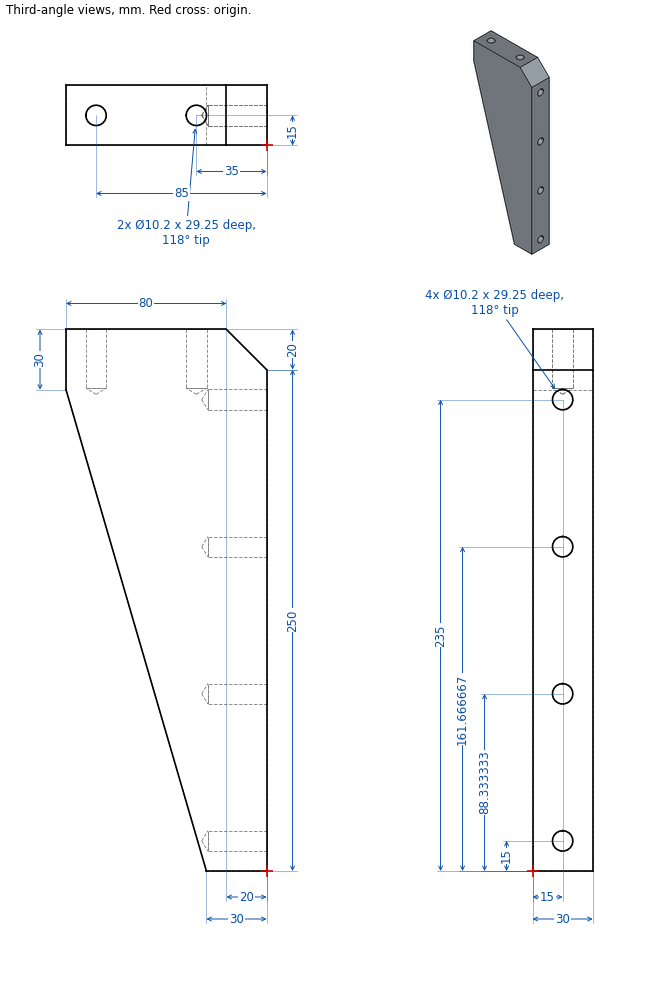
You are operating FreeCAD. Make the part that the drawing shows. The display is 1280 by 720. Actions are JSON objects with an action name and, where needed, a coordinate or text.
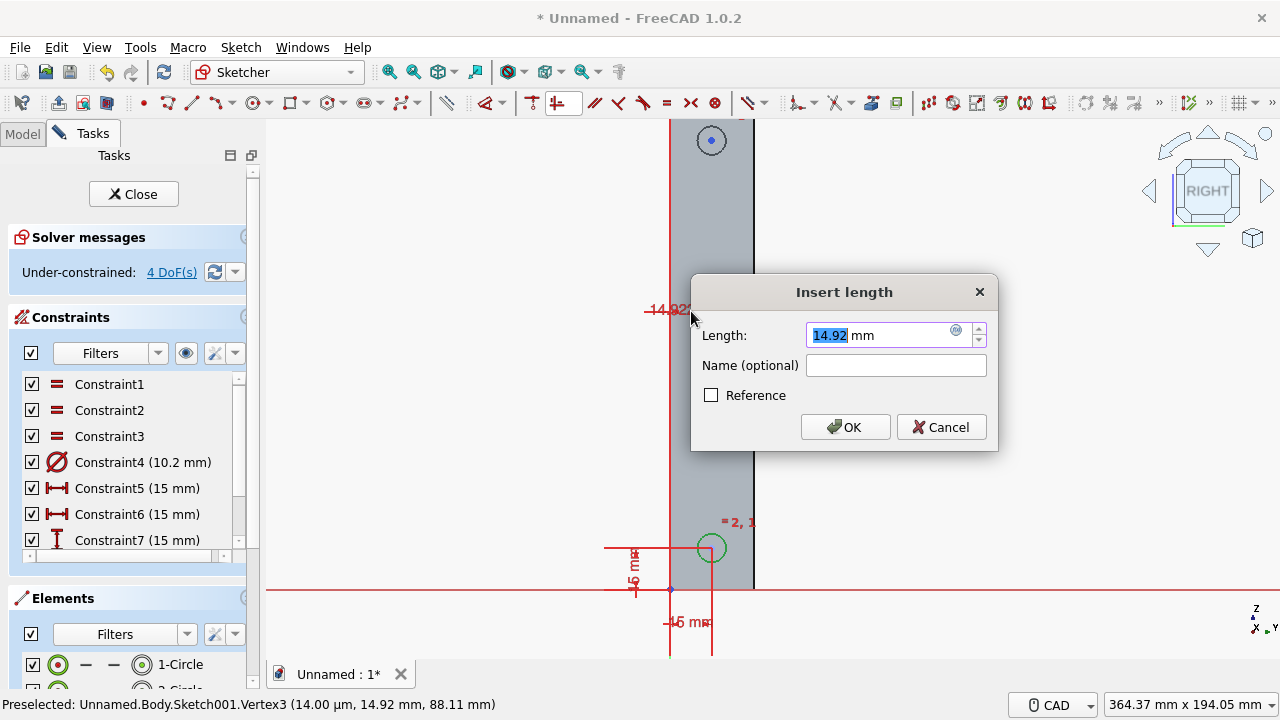
{"action": "type", "text": "15"}
{"action": "key", "text": "Return"}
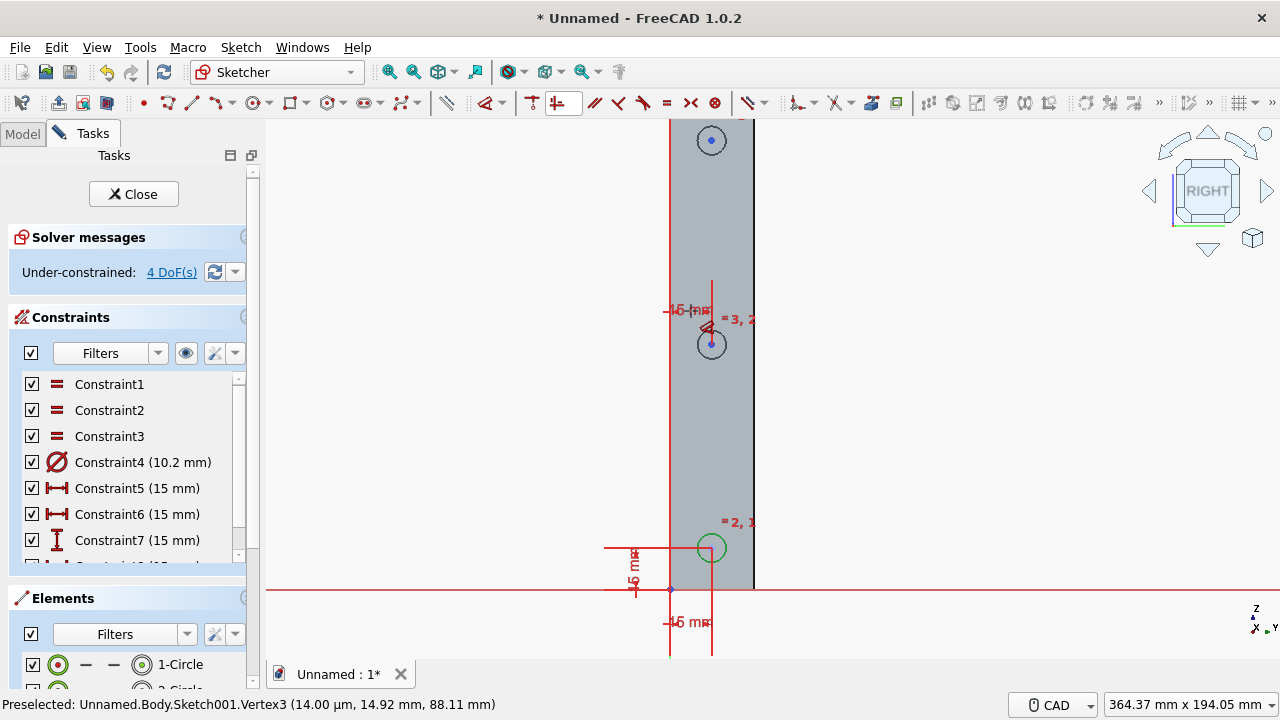
{"action": "scroll", "coordinate": [712, 551], "scroll_direction": "down", "scroll_amount": 3}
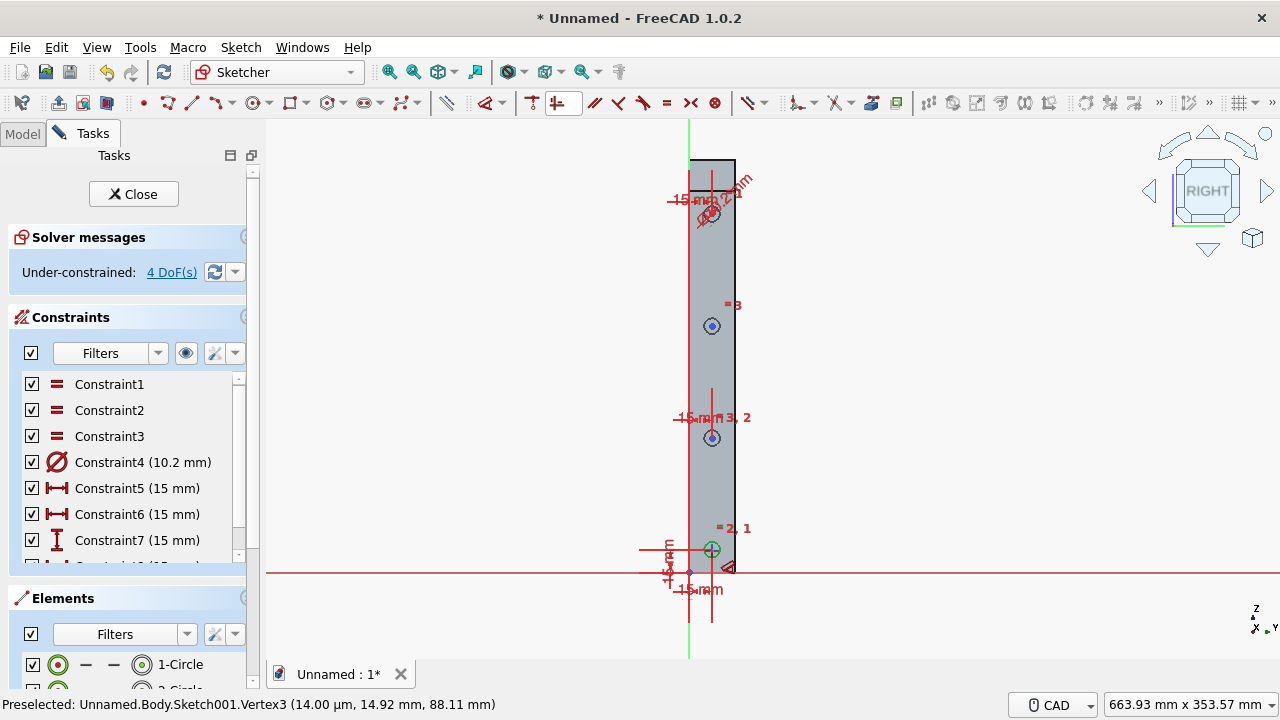
{"action": "scroll", "coordinate": [712, 326], "scroll_direction": "up", "scroll_amount": 3}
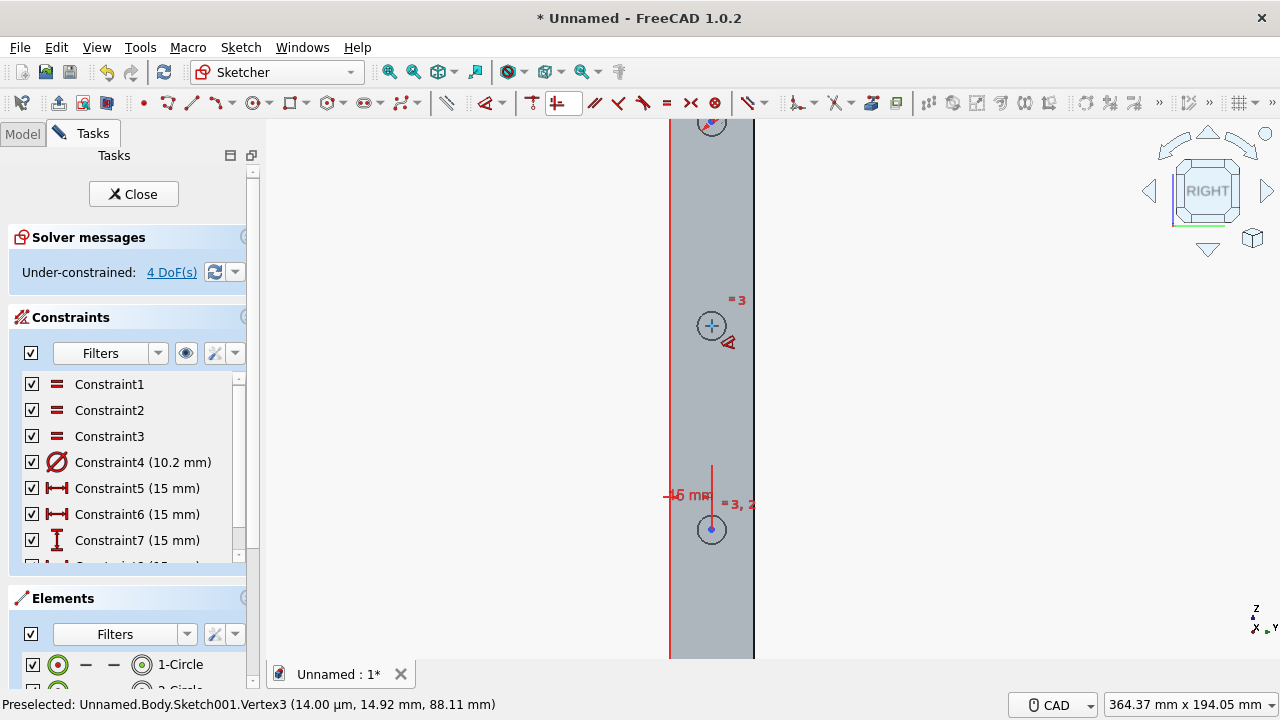
{"action": "left_click", "coordinate": [712, 326]}
{"action": "left_click", "coordinate": [691, 292]}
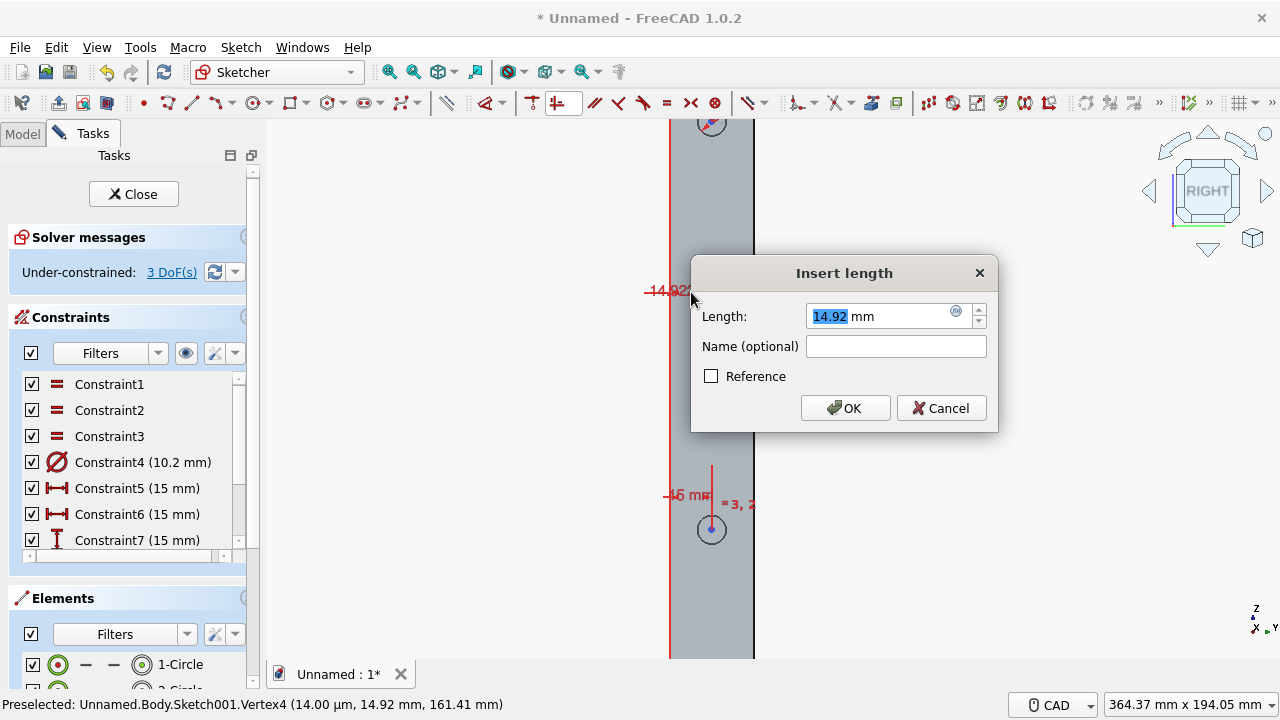
{"action": "type", "text": "15"}
{"action": "key", "text": "Return"}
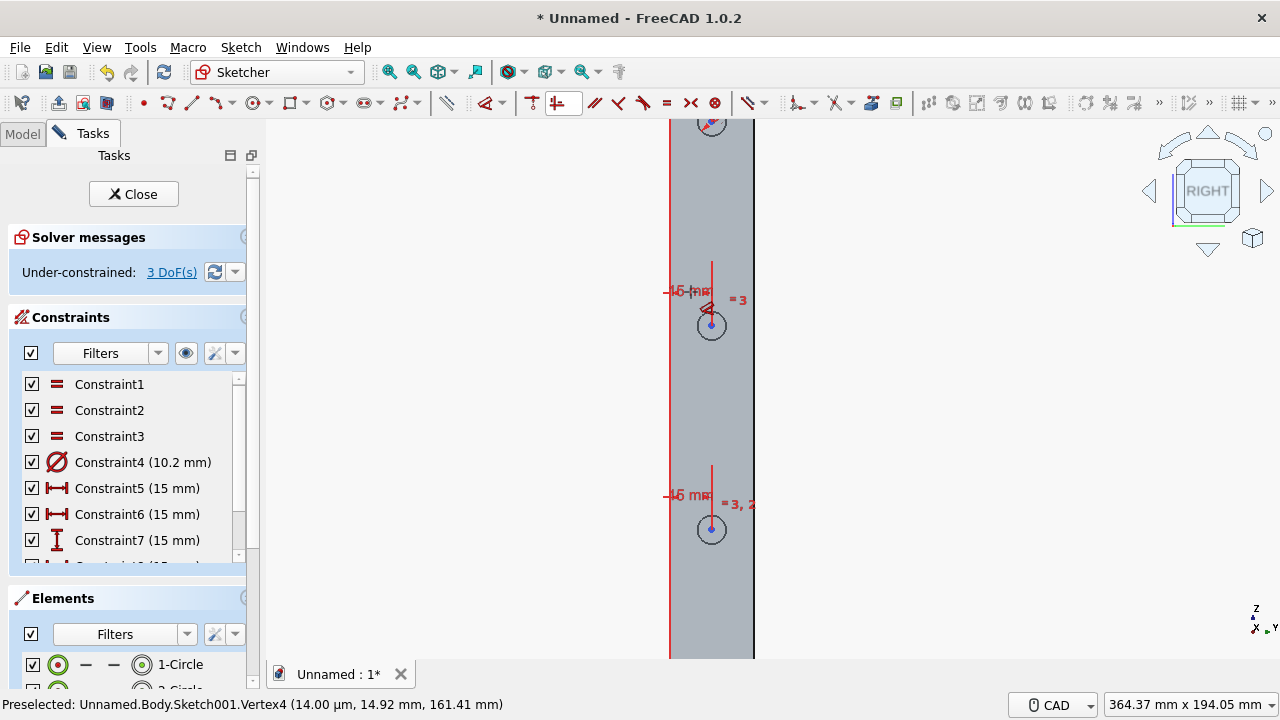
{"action": "scroll", "coordinate": [712, 326], "scroll_direction": "down", "scroll_amount": 3}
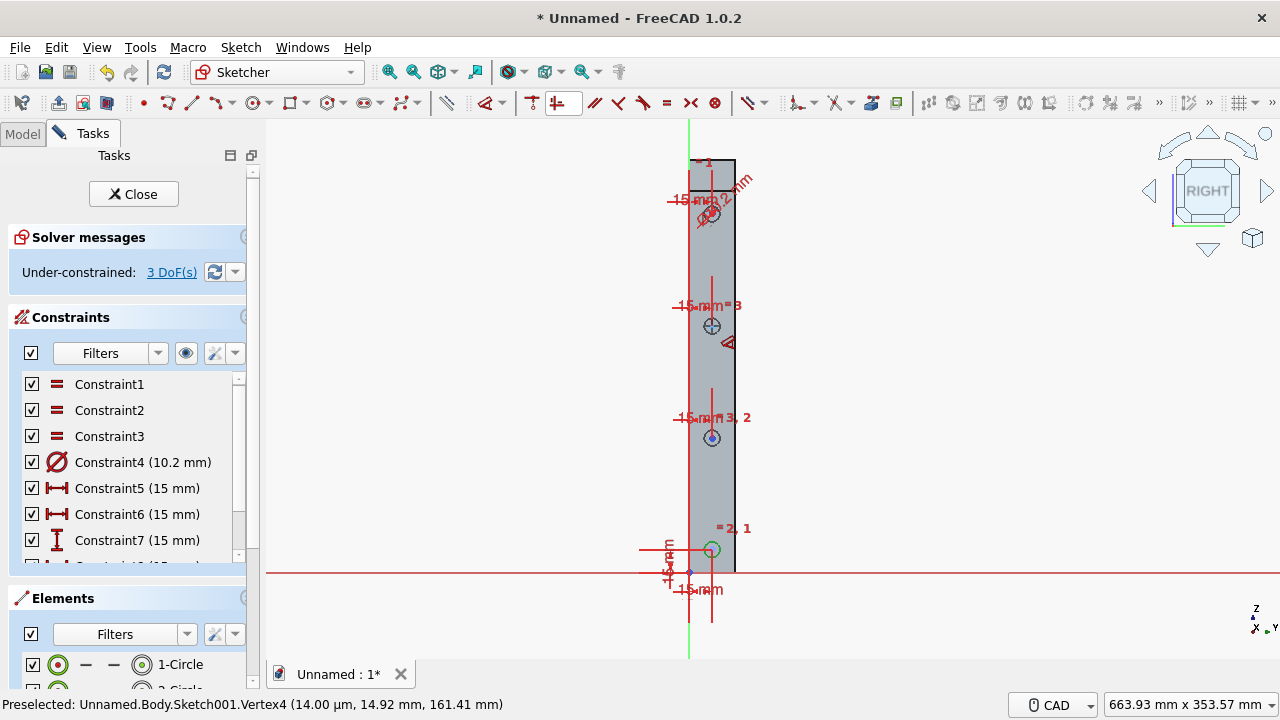
{"action": "left_click", "coordinate": [712, 214]}
{"action": "left_click", "coordinate": [655, 393]}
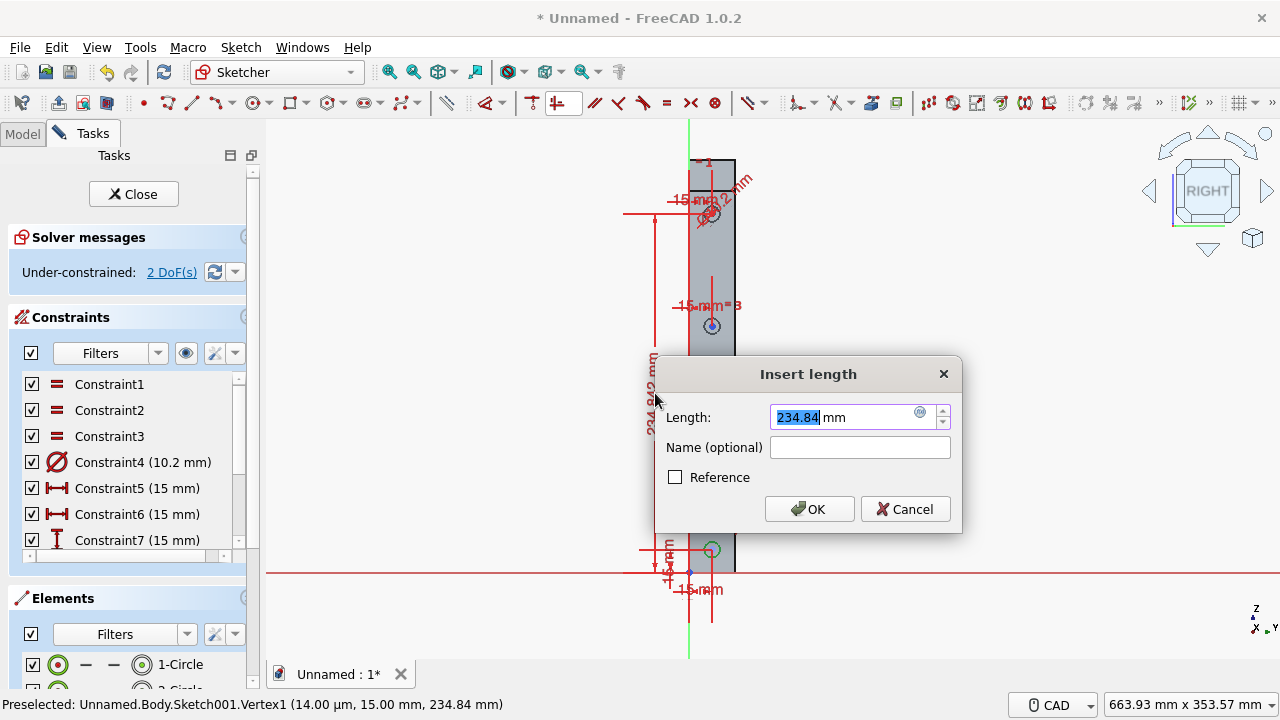
{"action": "type", "text": "235"}
{"action": "key", "text": "Return"}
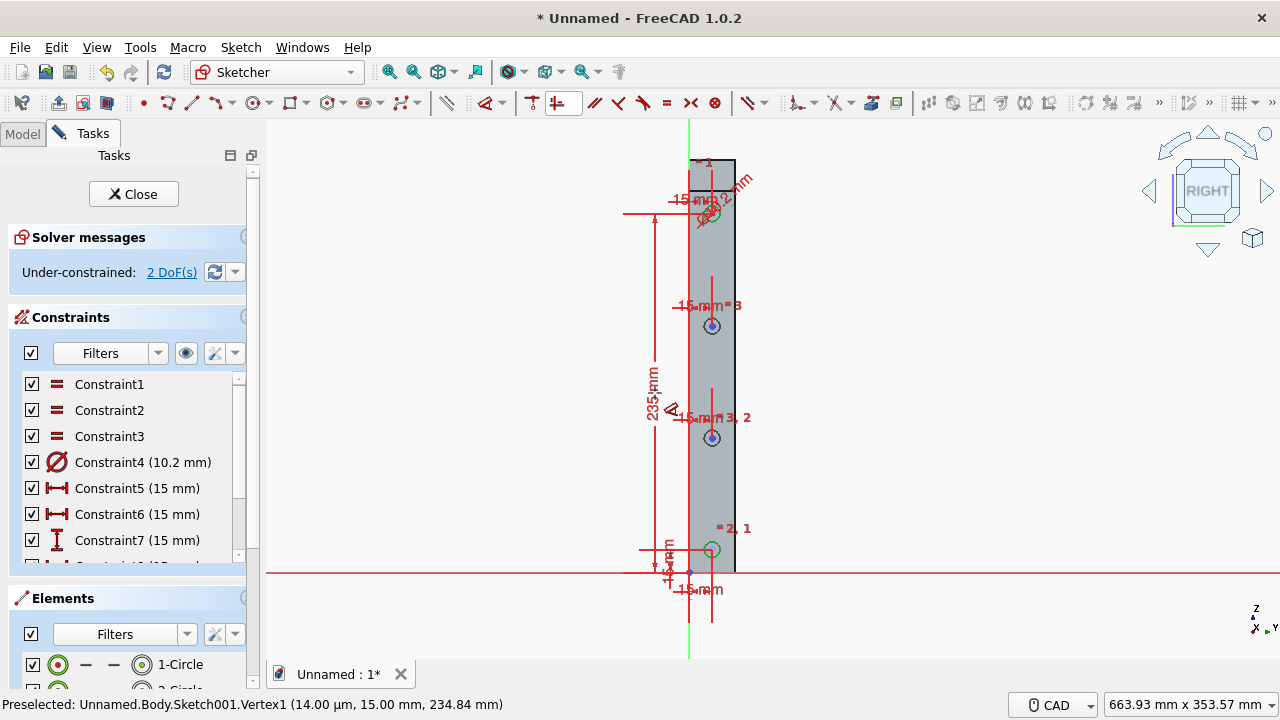
{"action": "left_click", "coordinate": [712, 438]}
{"action": "left_click", "coordinate": [655, 505]}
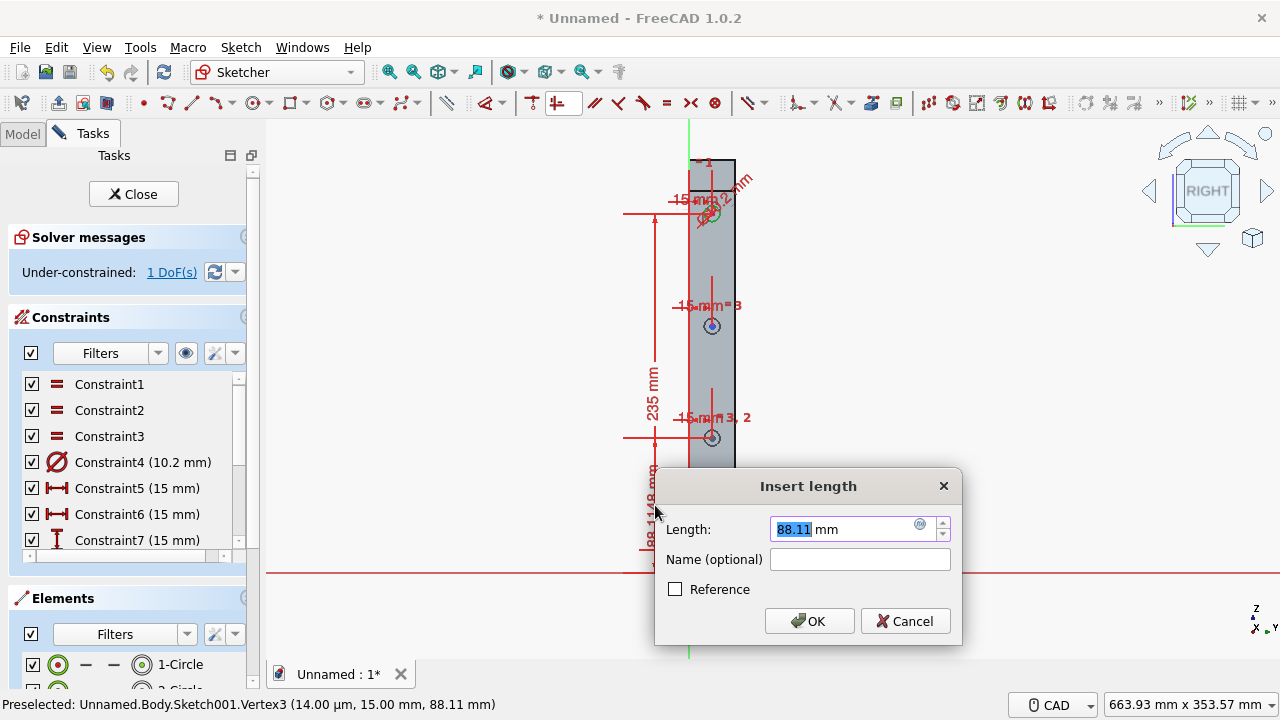
{"action": "type", "text": "88.333333"}
{"action": "key", "text": "Return"}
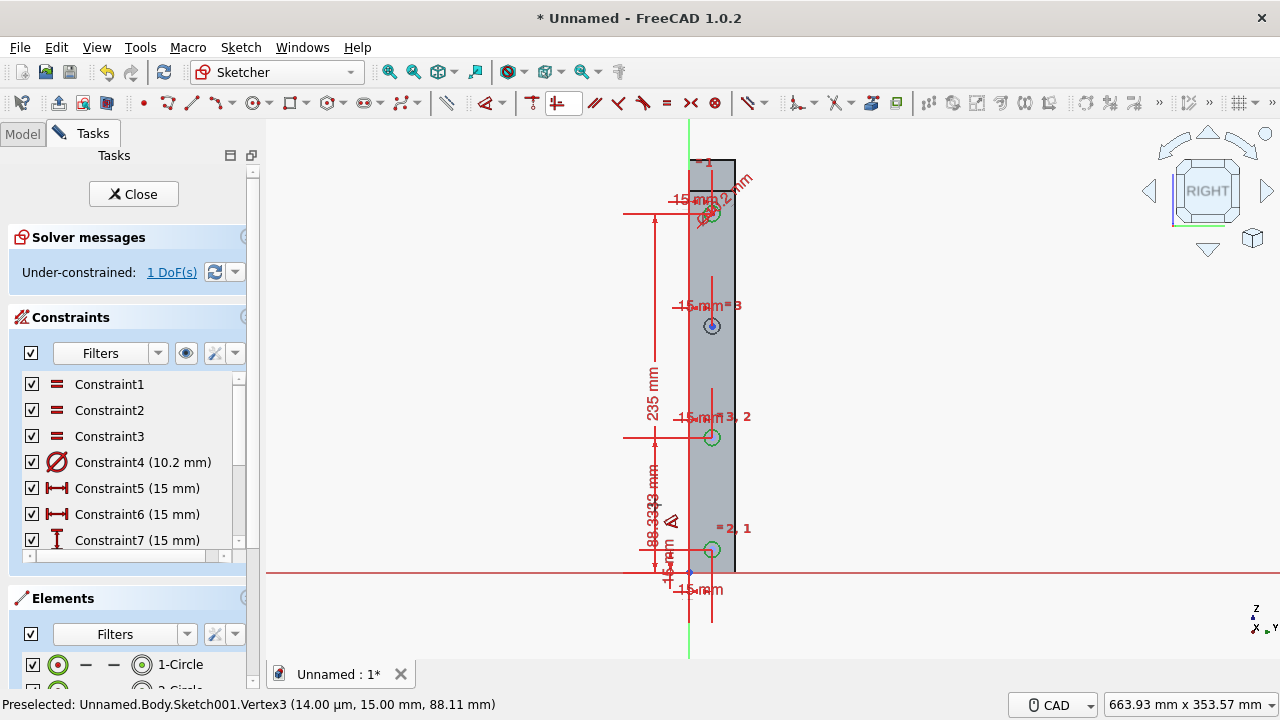
{"action": "left_click", "coordinate": [712, 326]}
{"action": "left_click", "coordinate": [655, 449]}